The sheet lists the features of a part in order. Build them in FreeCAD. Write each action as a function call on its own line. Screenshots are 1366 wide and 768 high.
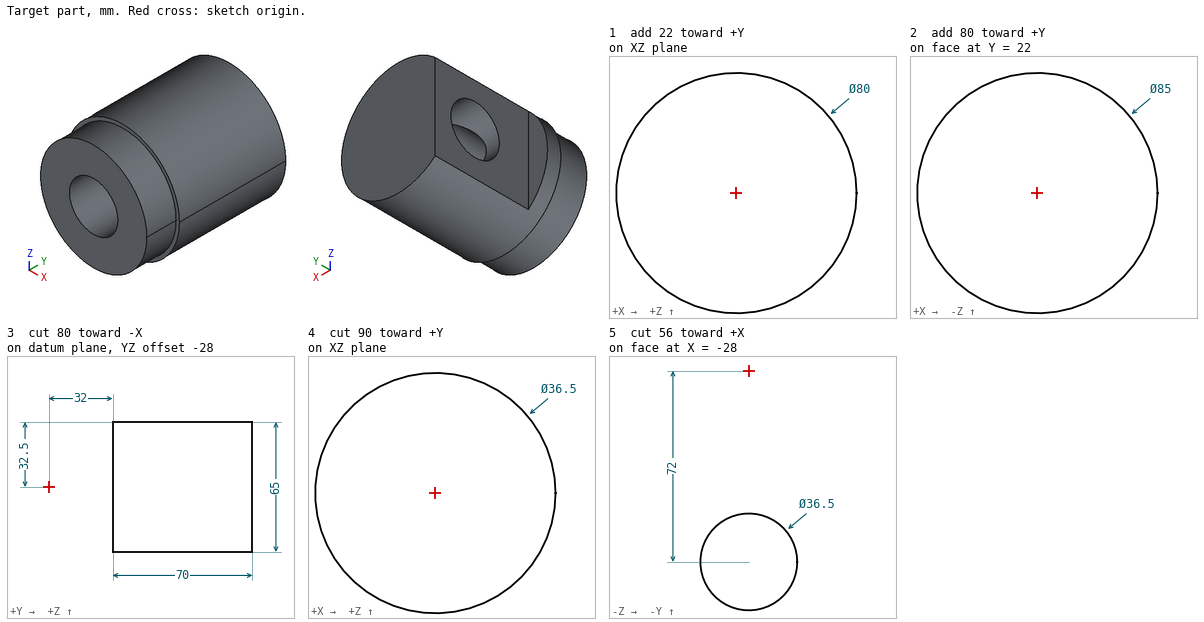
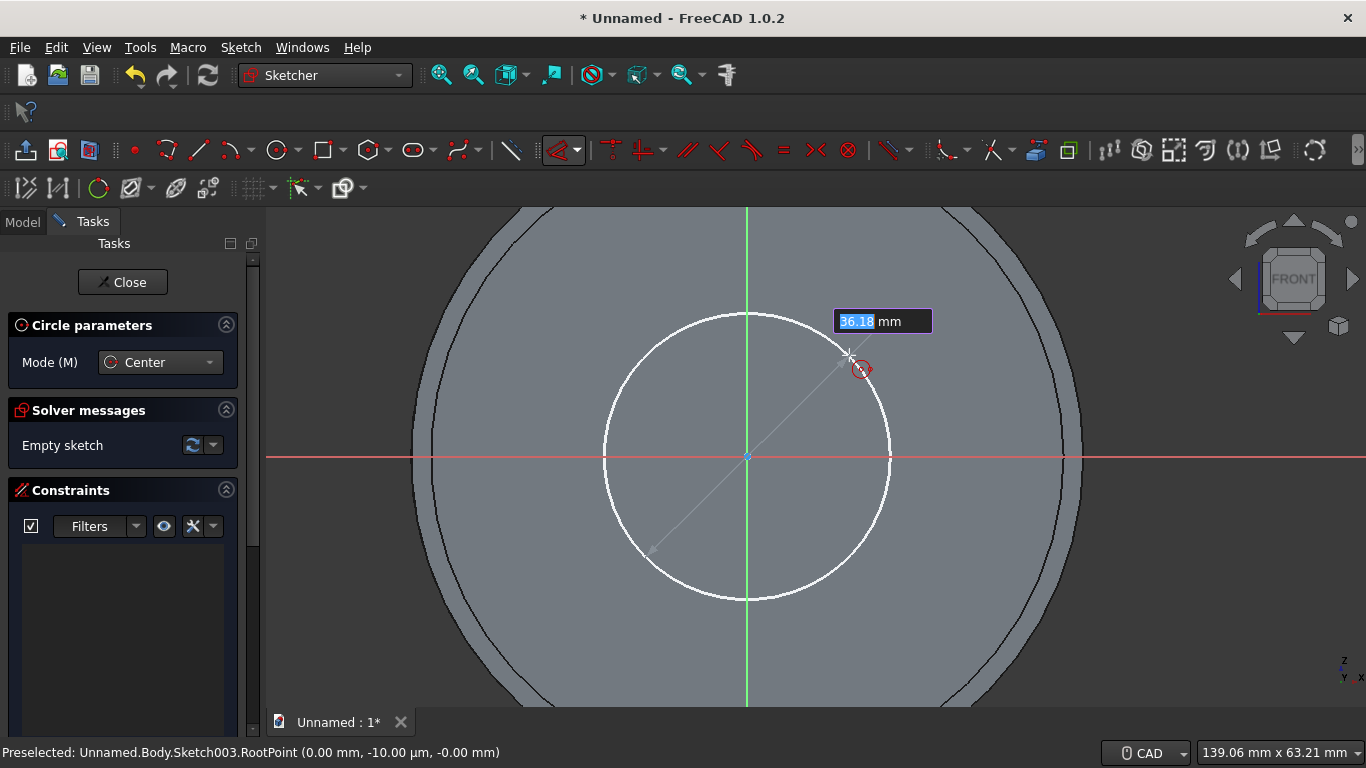
text(36.5)
key(Return)
key(Escape)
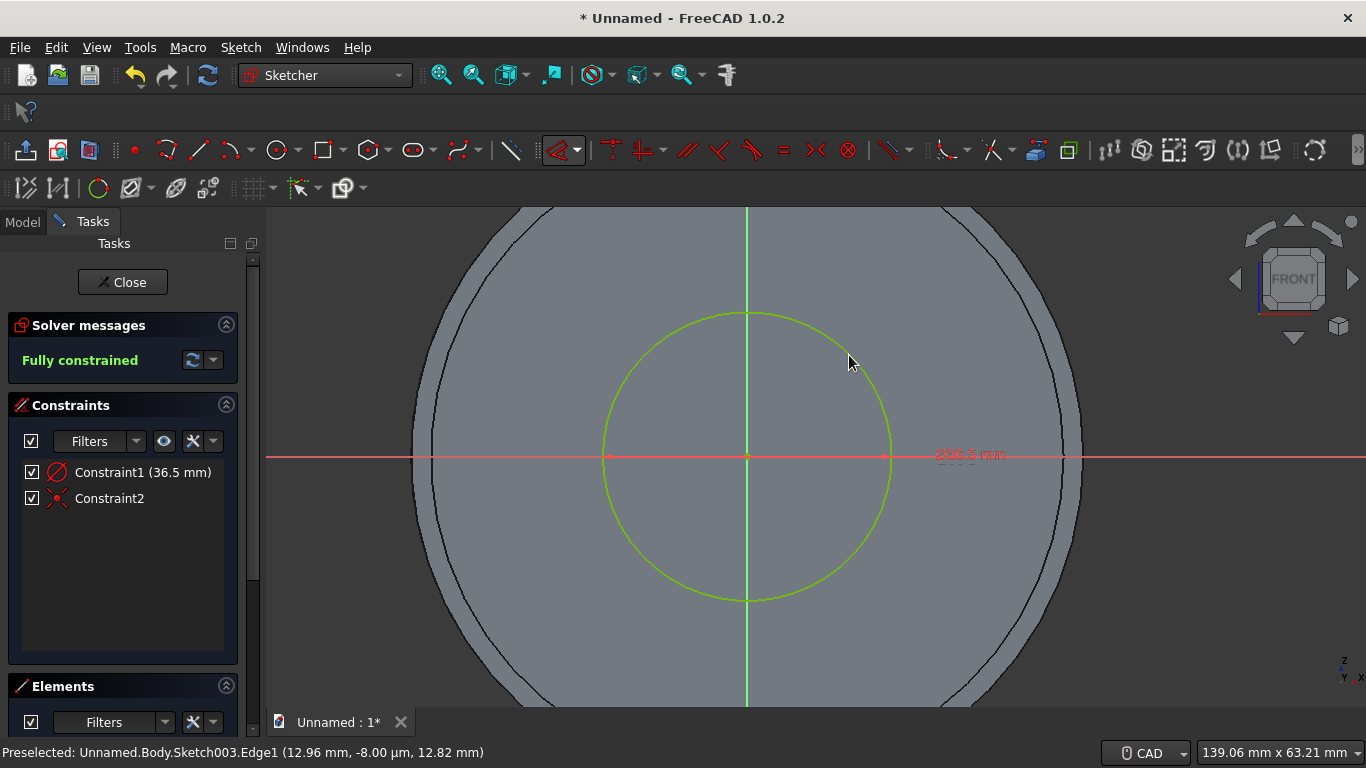
click(123, 282)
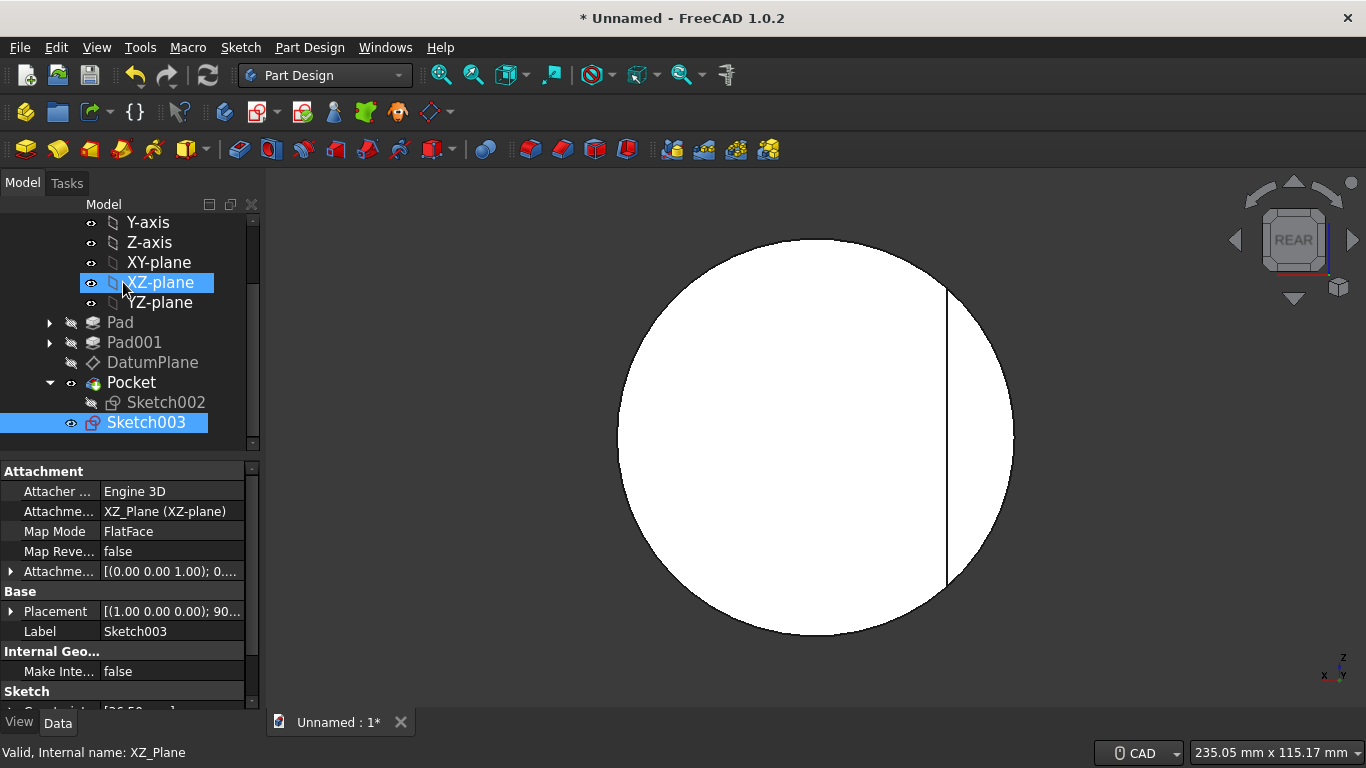
click(240, 150)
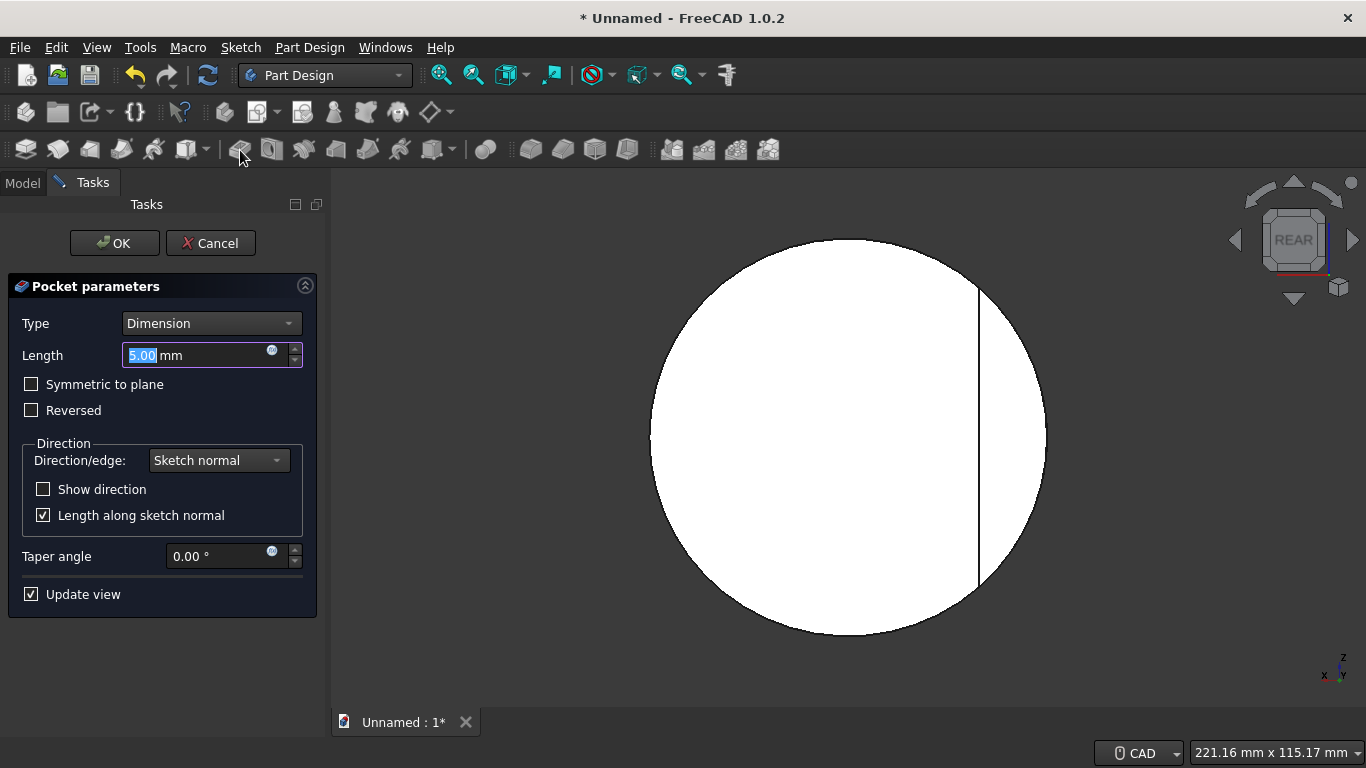
text(90)
key(Tab)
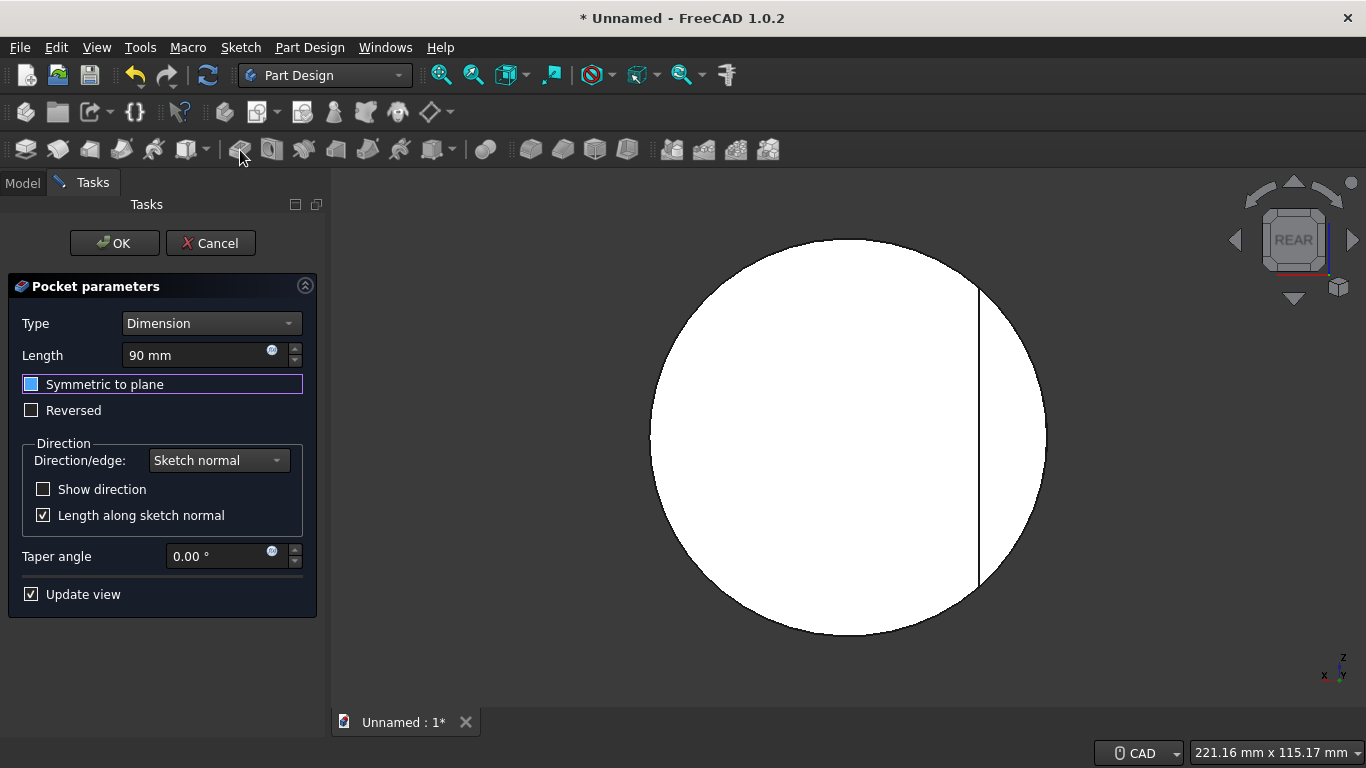
click(115, 243)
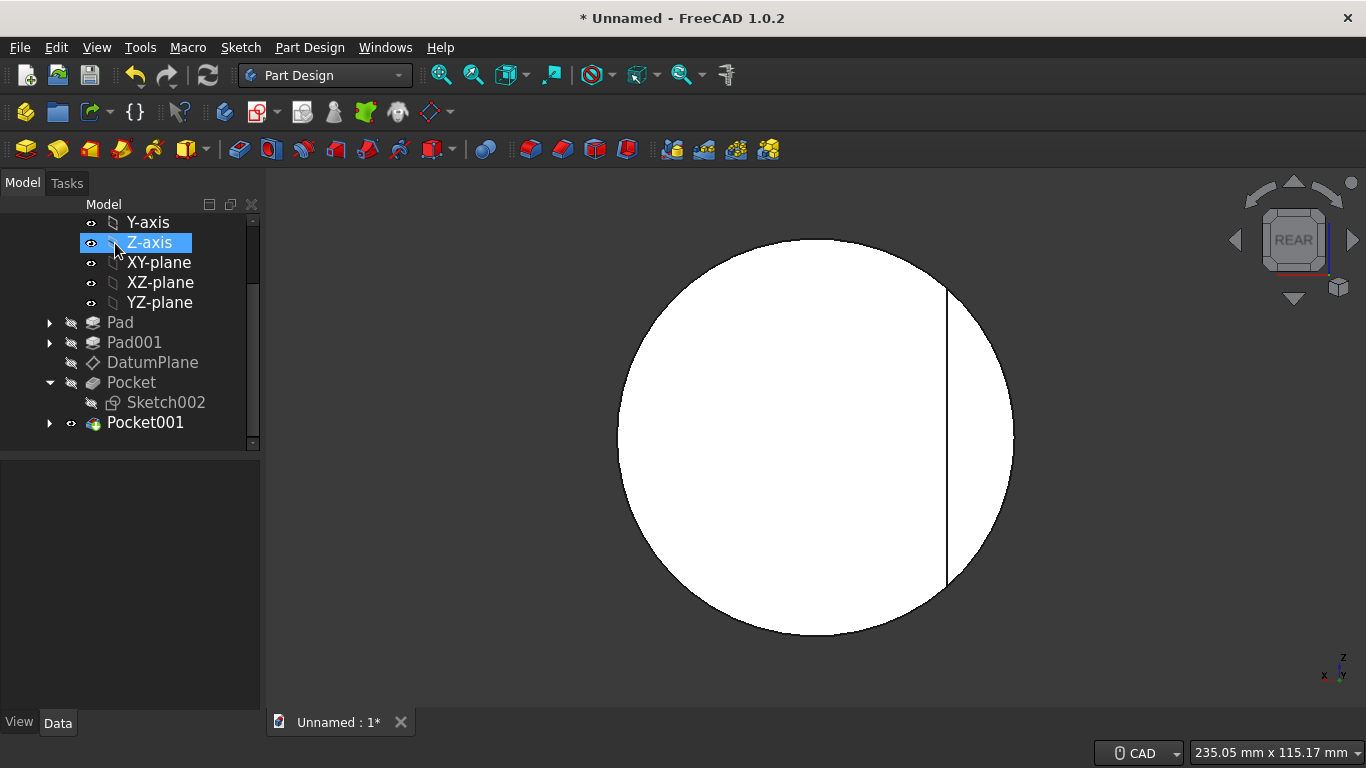
key(6)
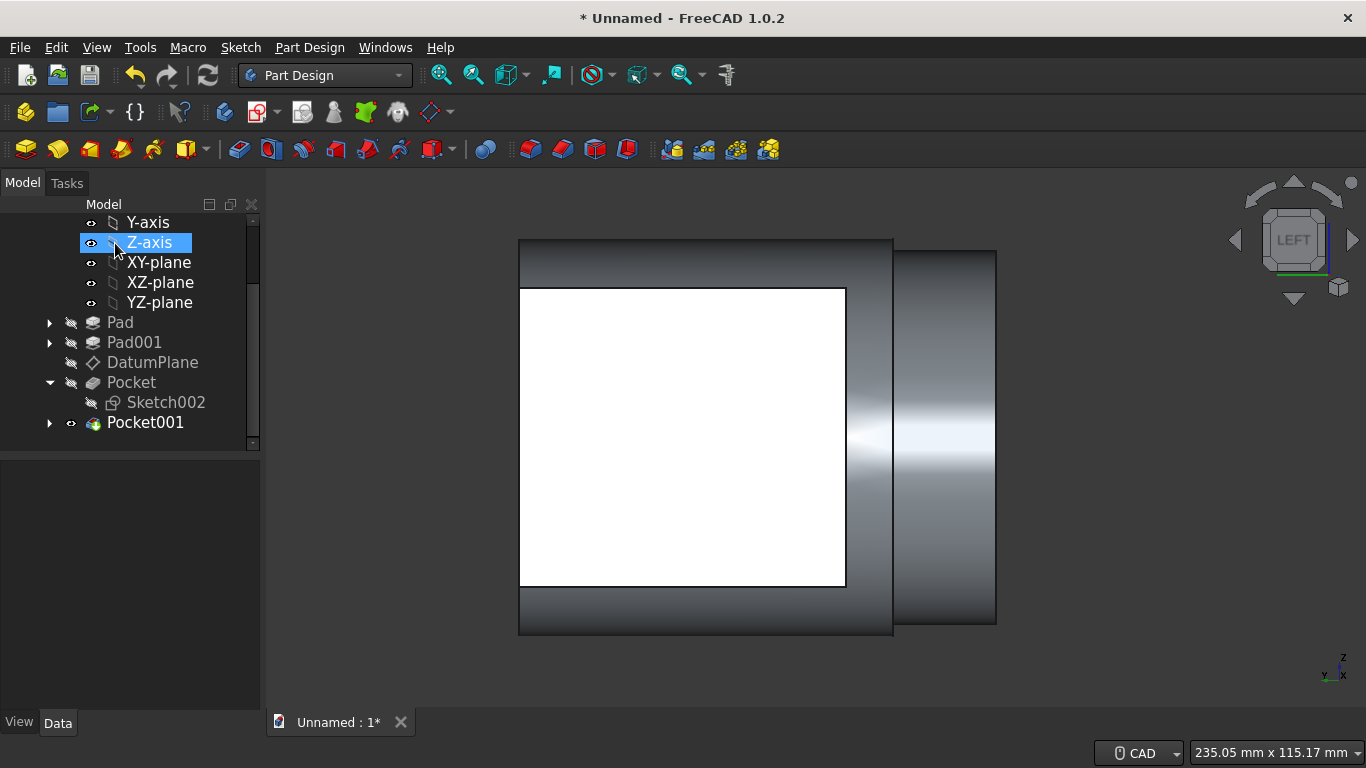
click(683, 437)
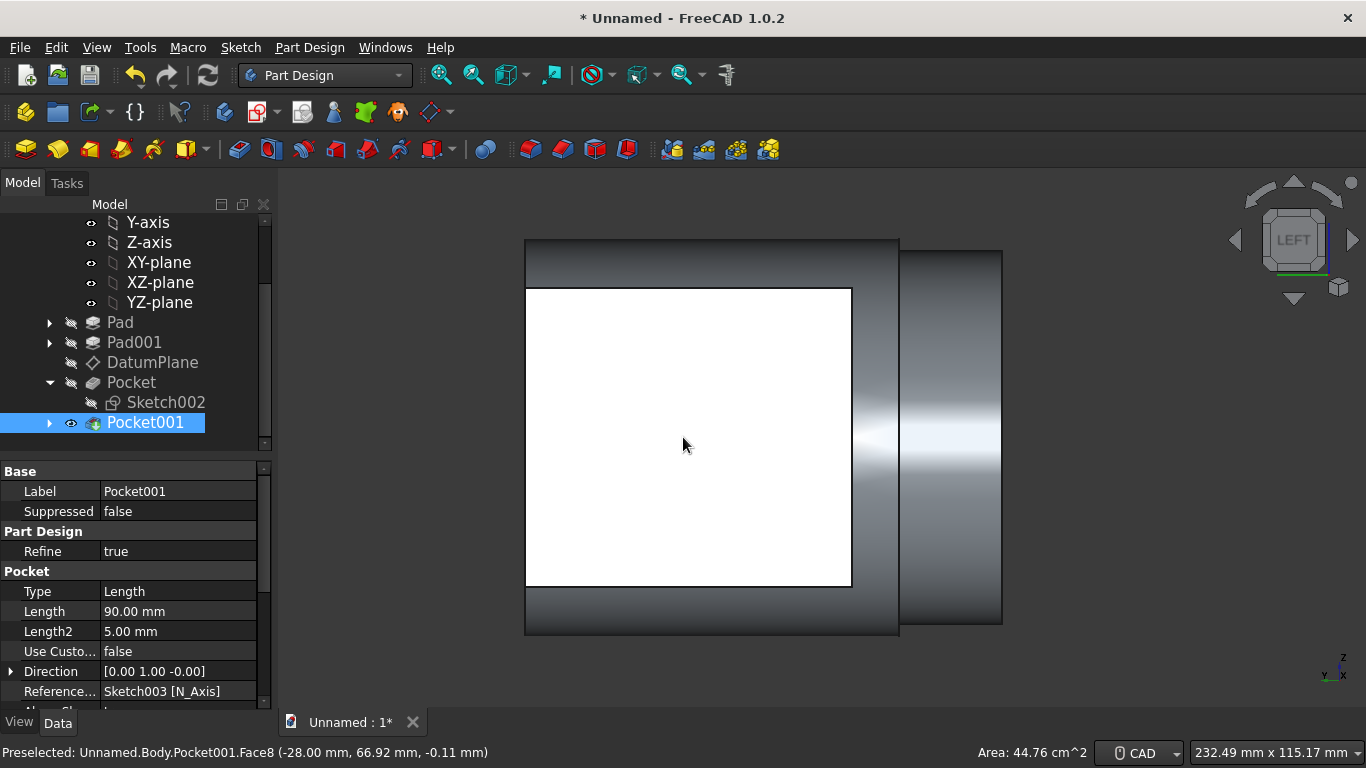
click(258, 112)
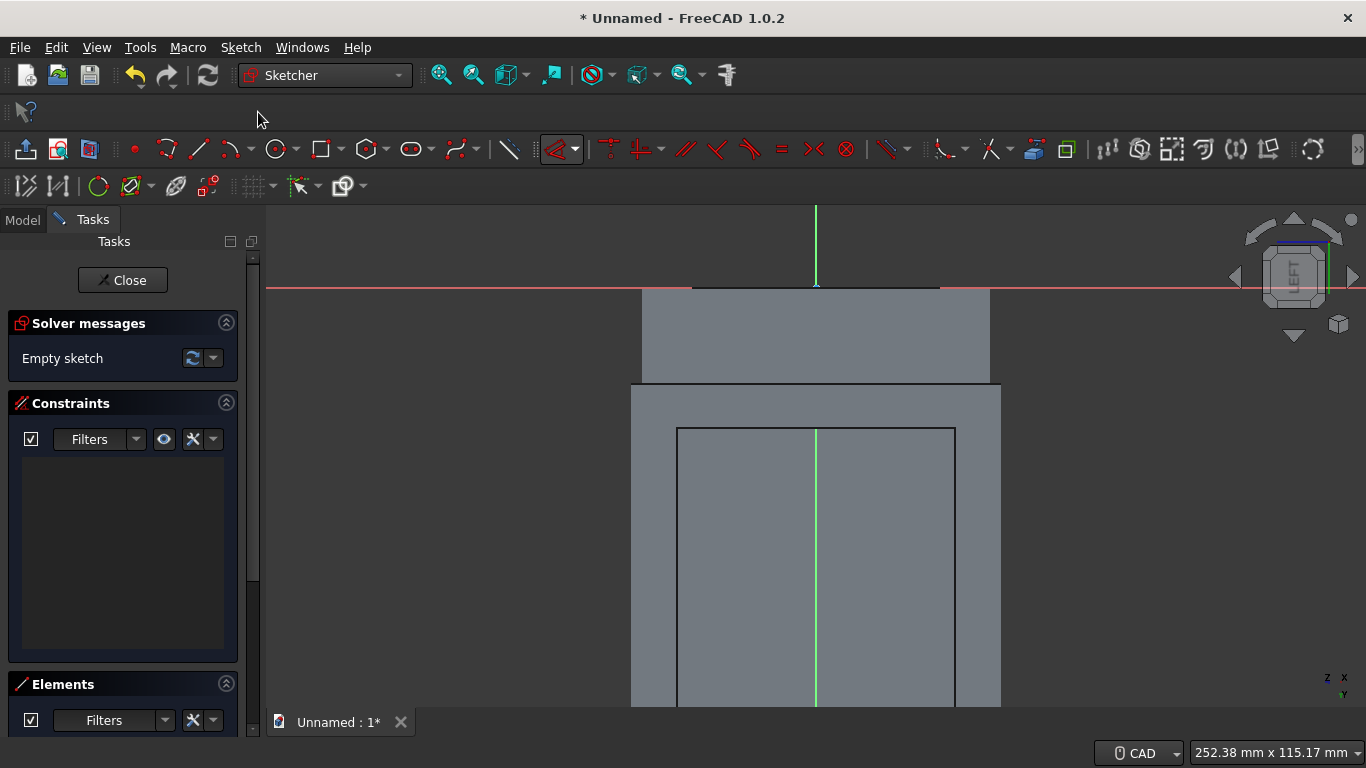
scroll(438, 326, down, 1)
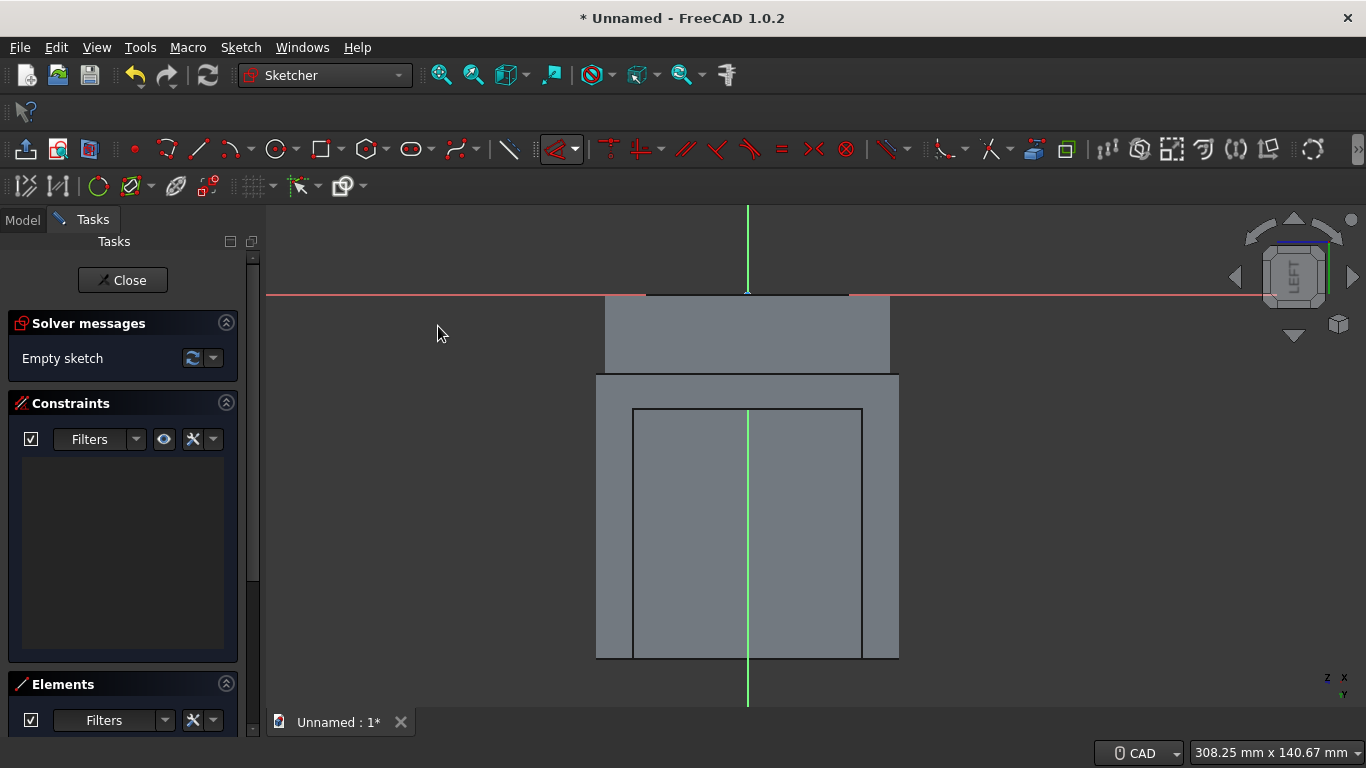
click(276, 150)